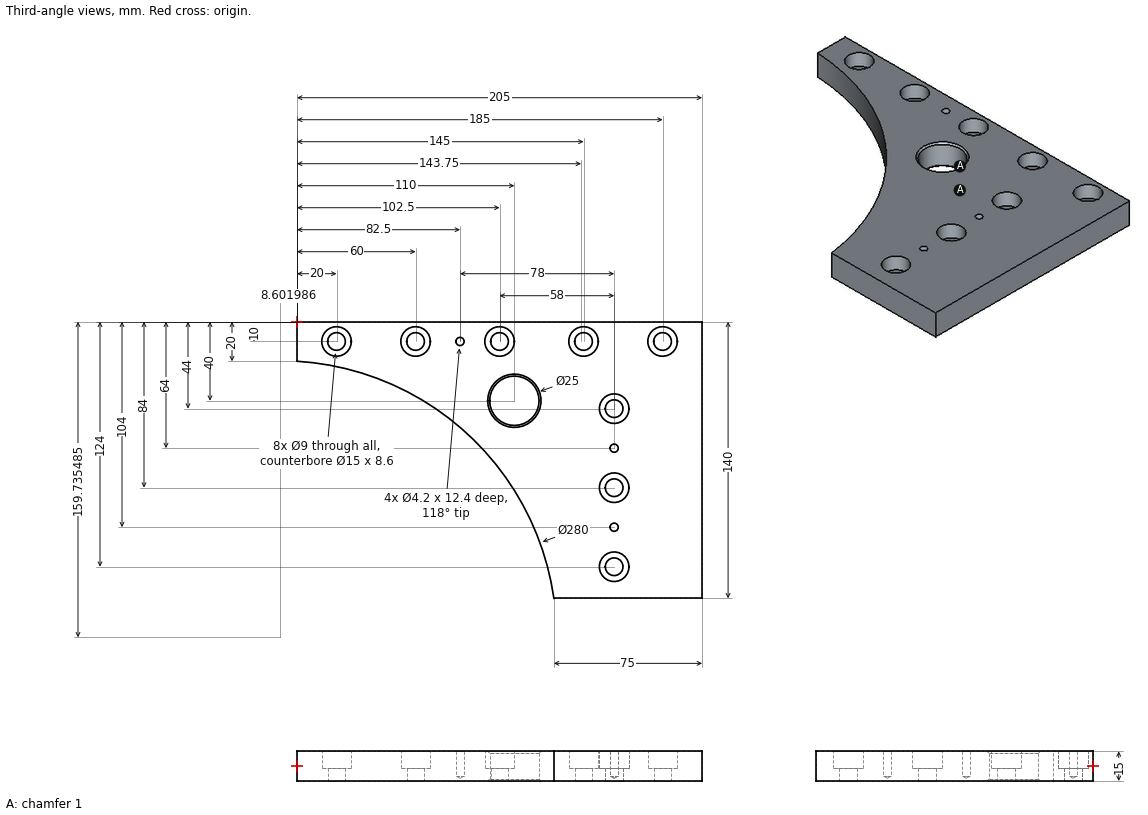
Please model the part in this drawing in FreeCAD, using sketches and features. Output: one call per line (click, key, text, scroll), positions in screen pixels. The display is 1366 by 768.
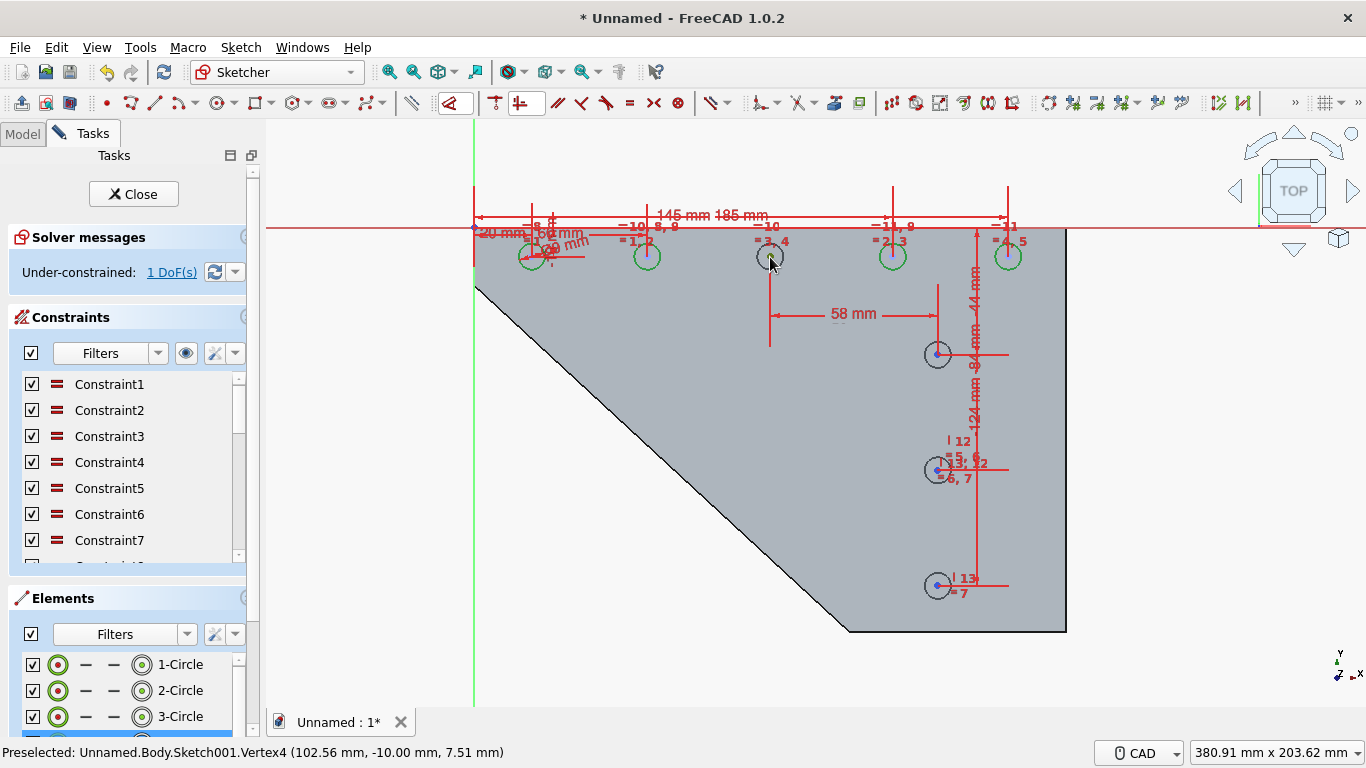
key(l)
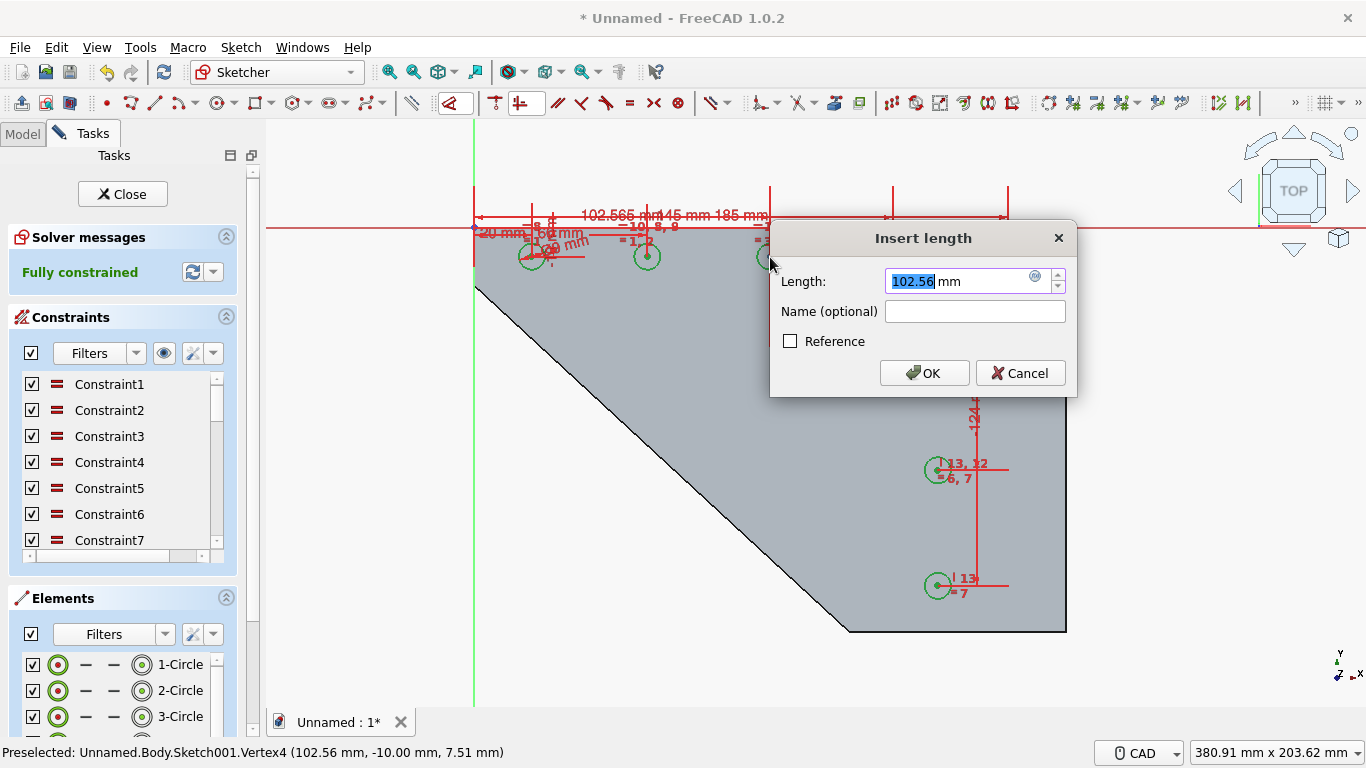
text(102.5)
key(Return)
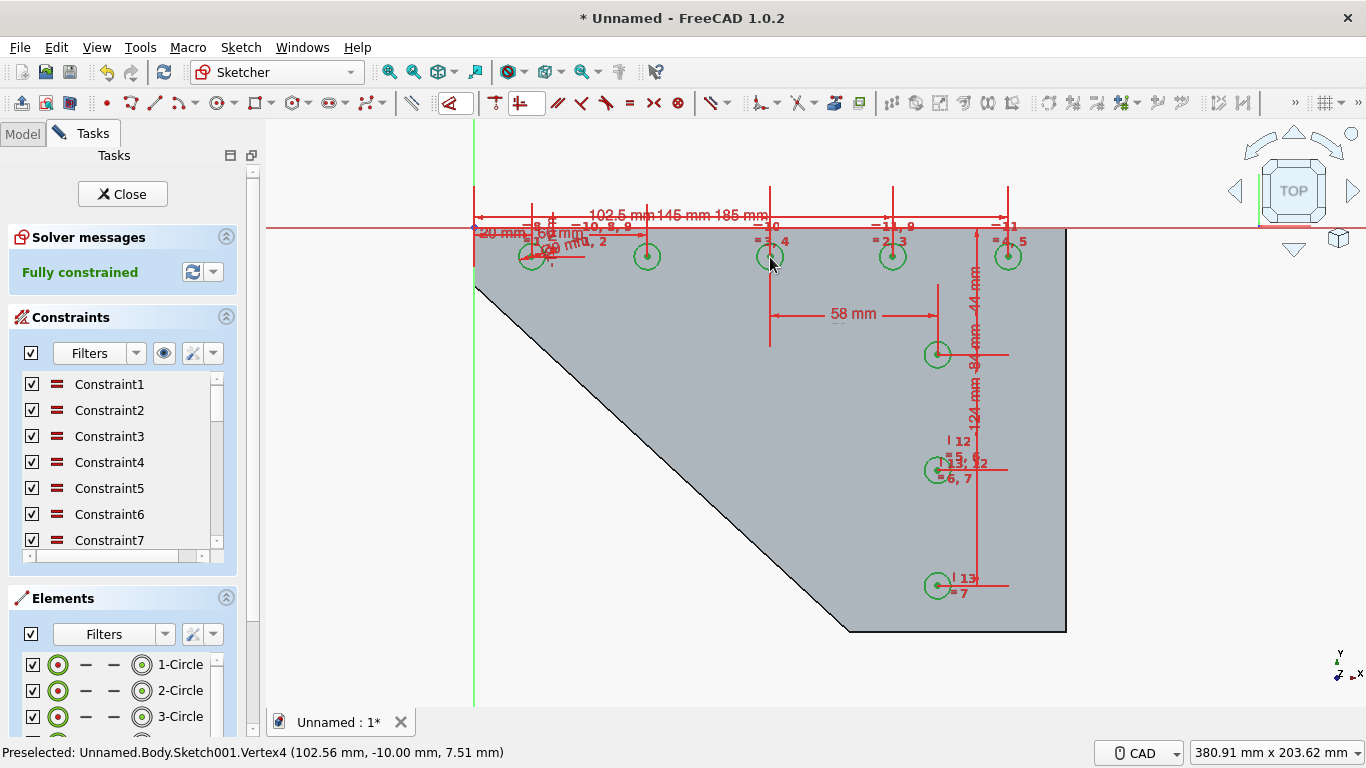
click(123, 194)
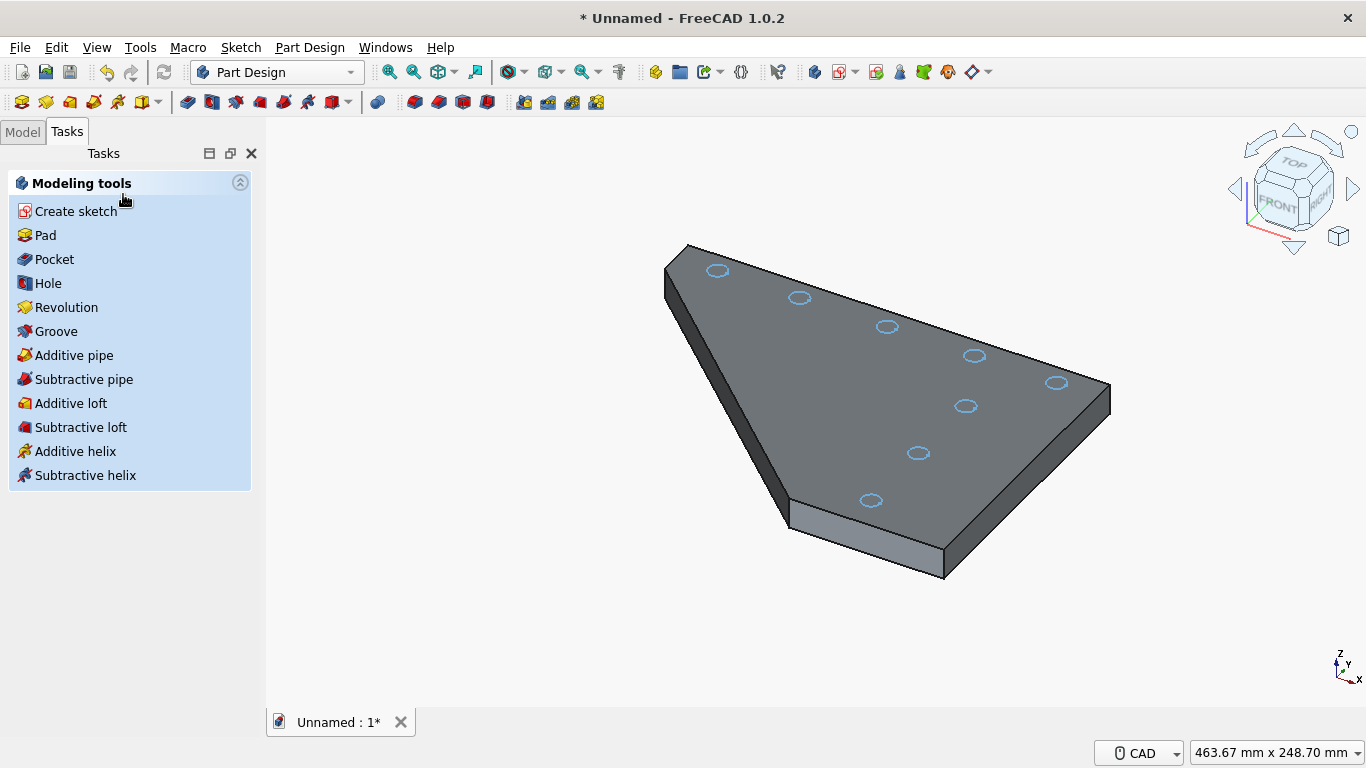
click(212, 102)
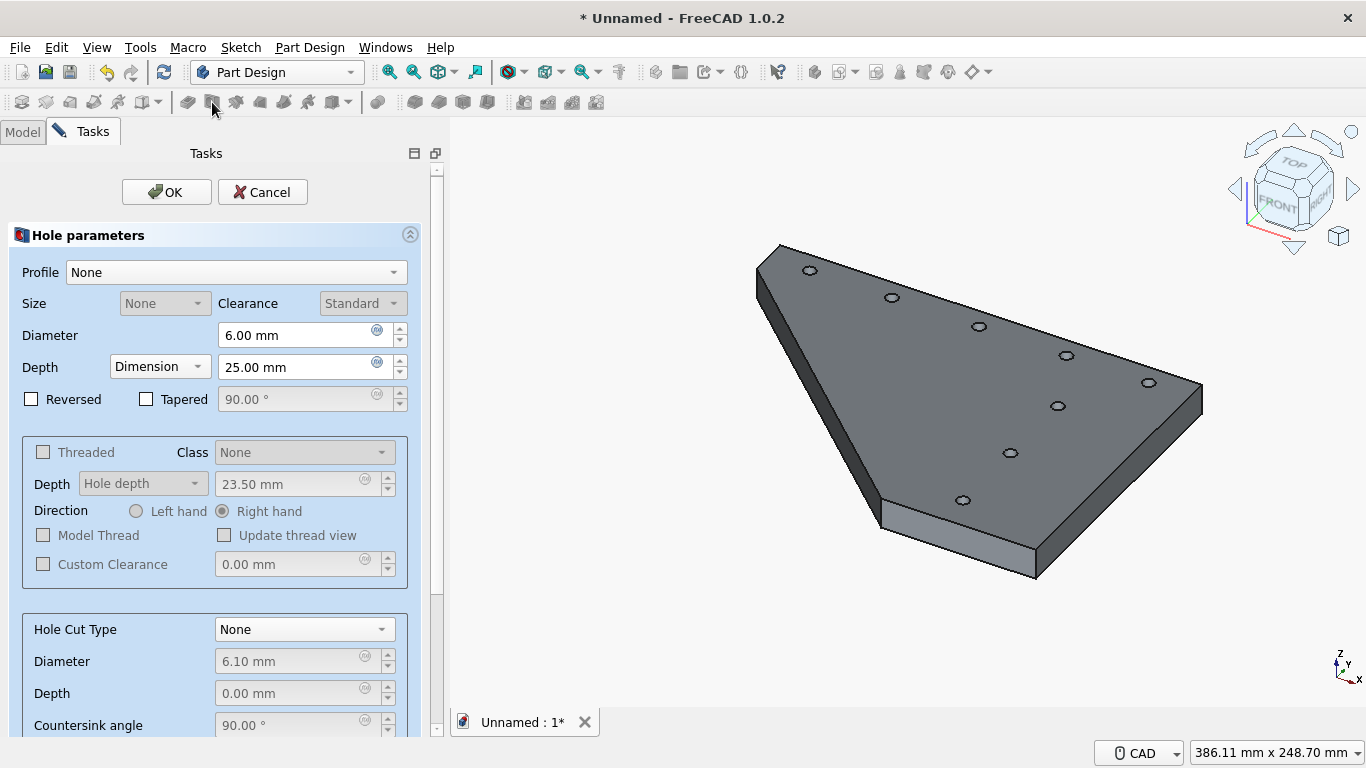
triple_click(305, 335)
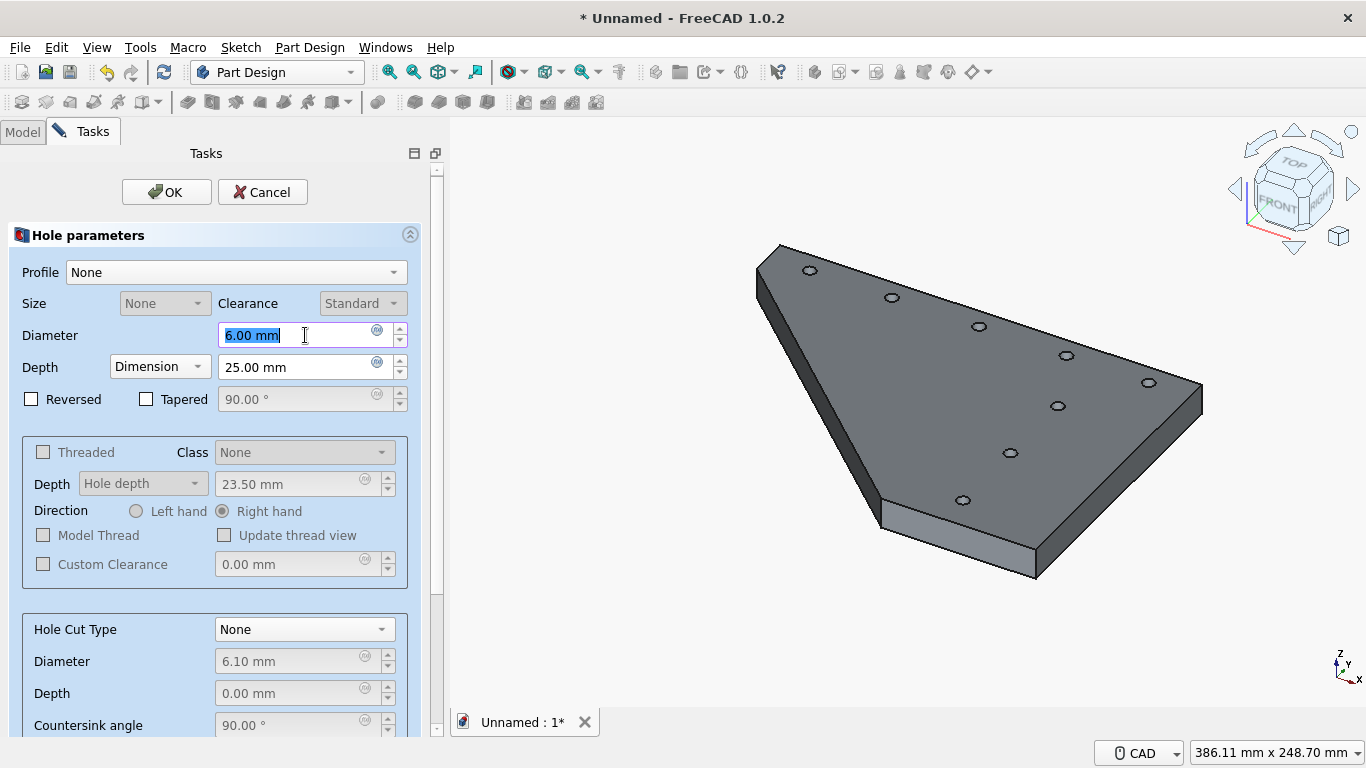
text(9)
key(Tab)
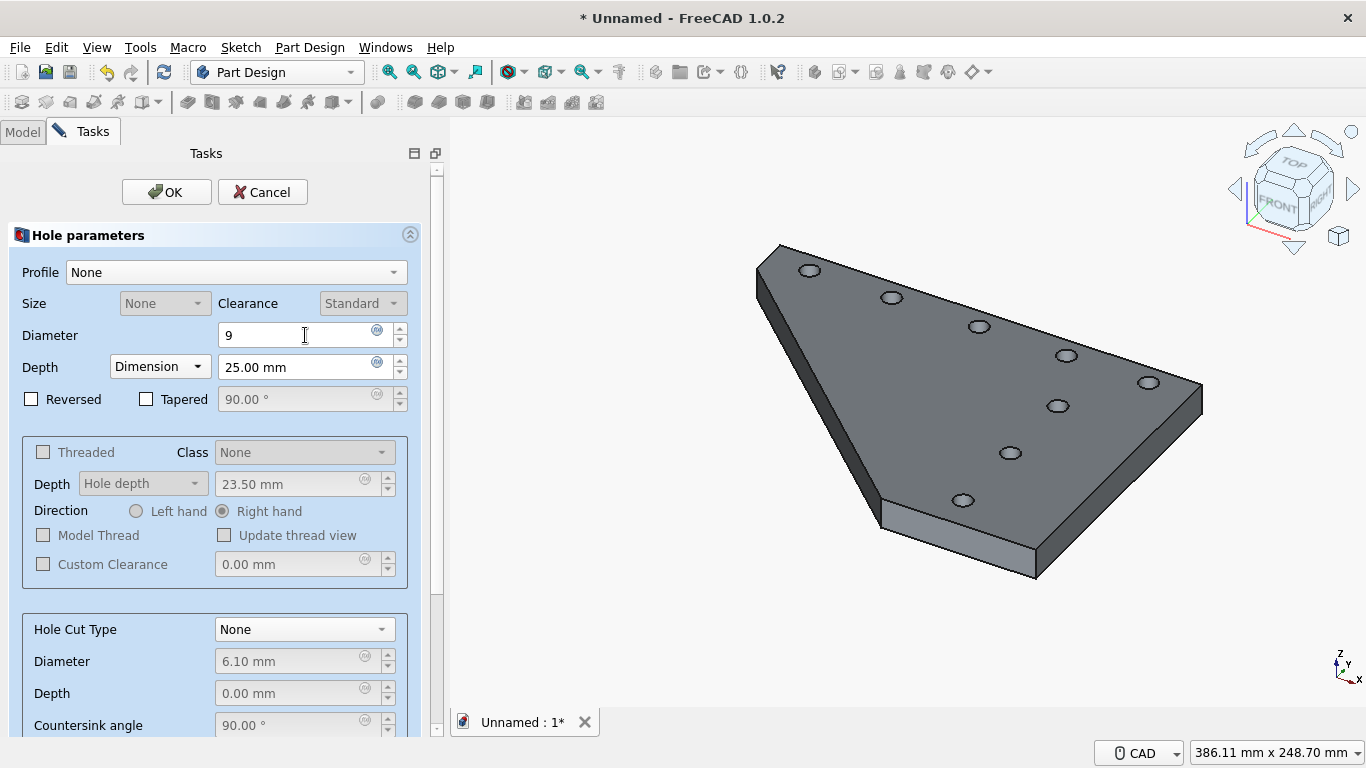
click(161, 366)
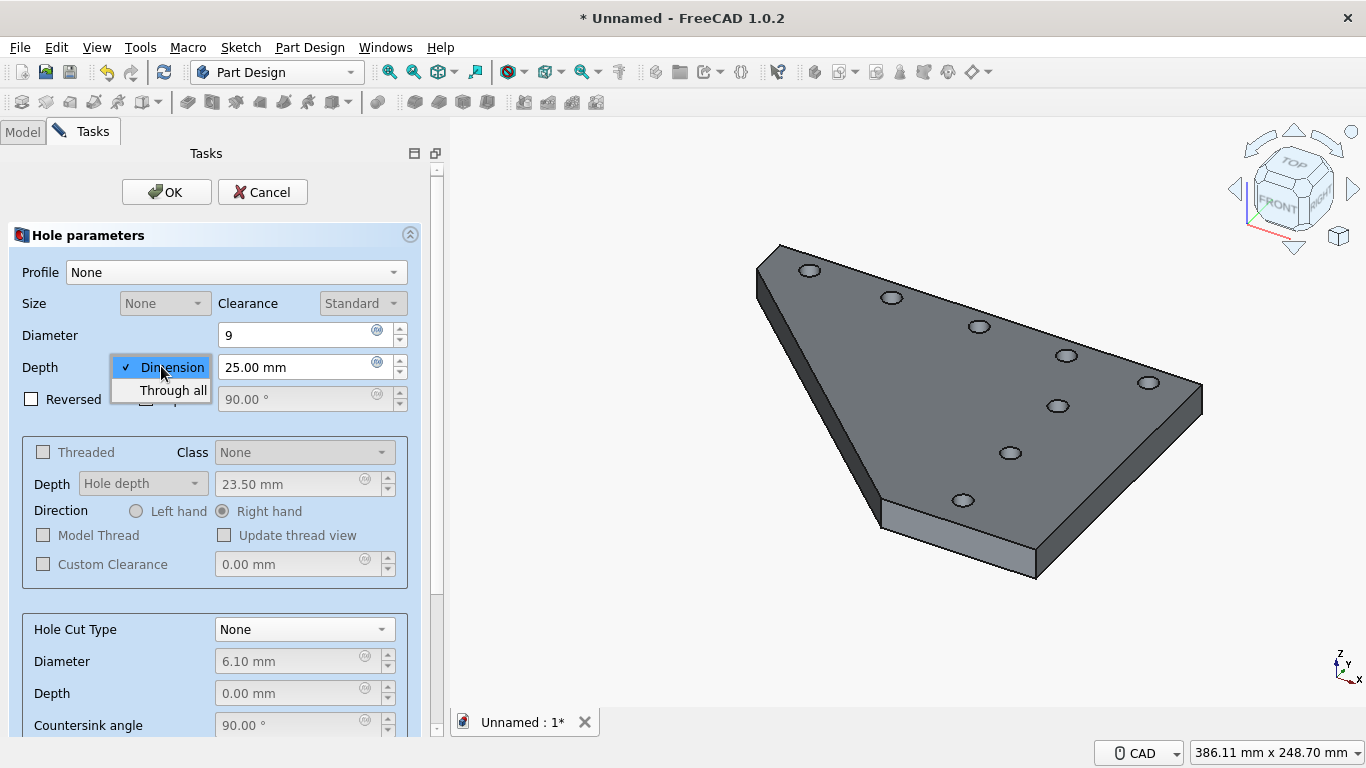
click(160, 390)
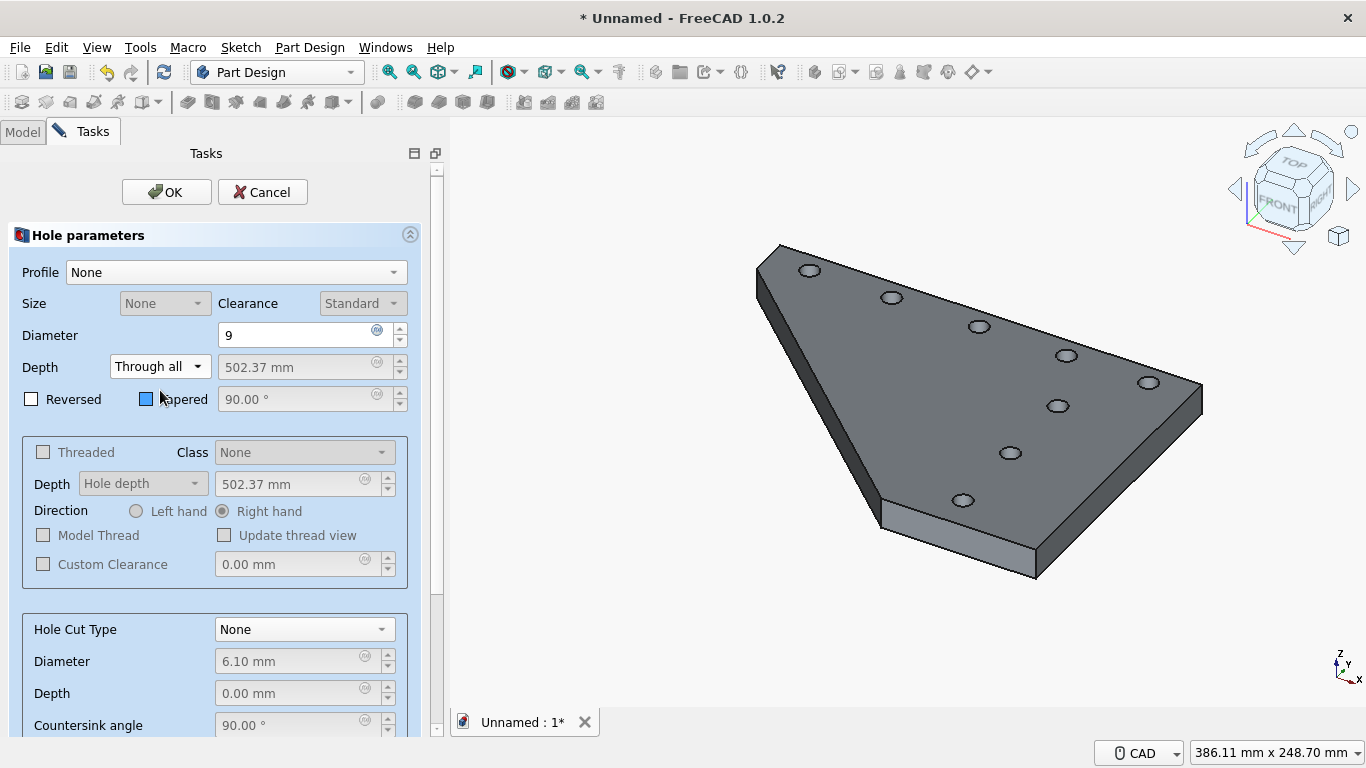
click(306, 630)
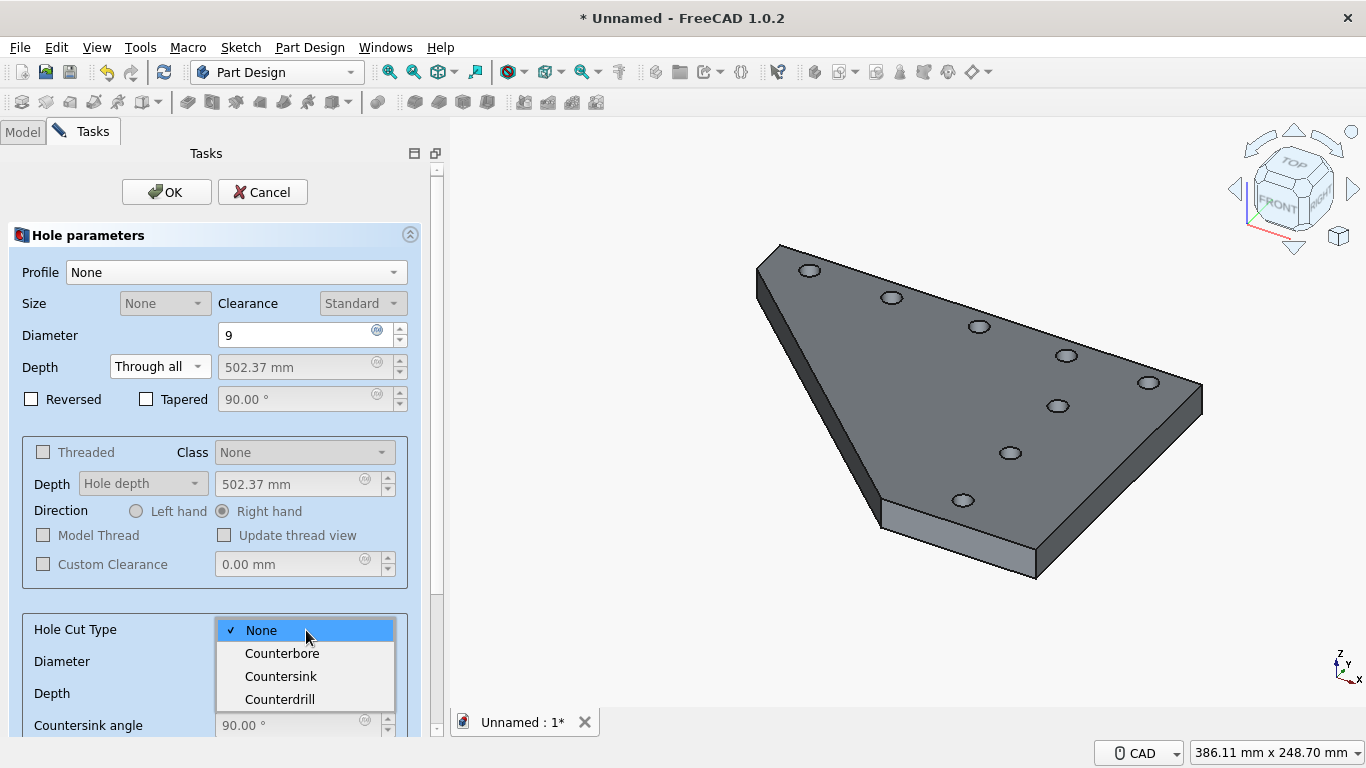
click(304, 654)